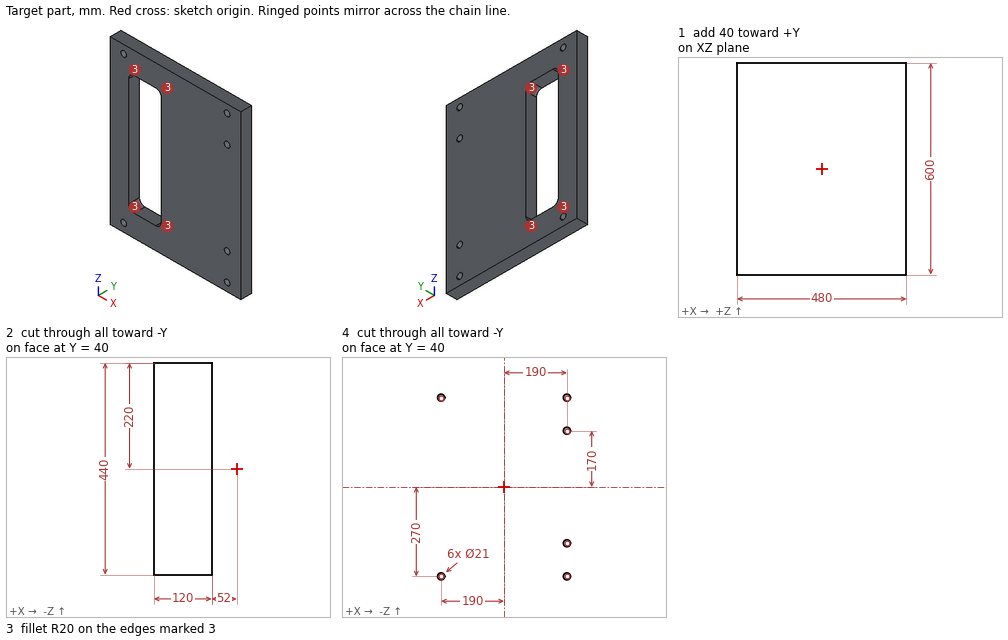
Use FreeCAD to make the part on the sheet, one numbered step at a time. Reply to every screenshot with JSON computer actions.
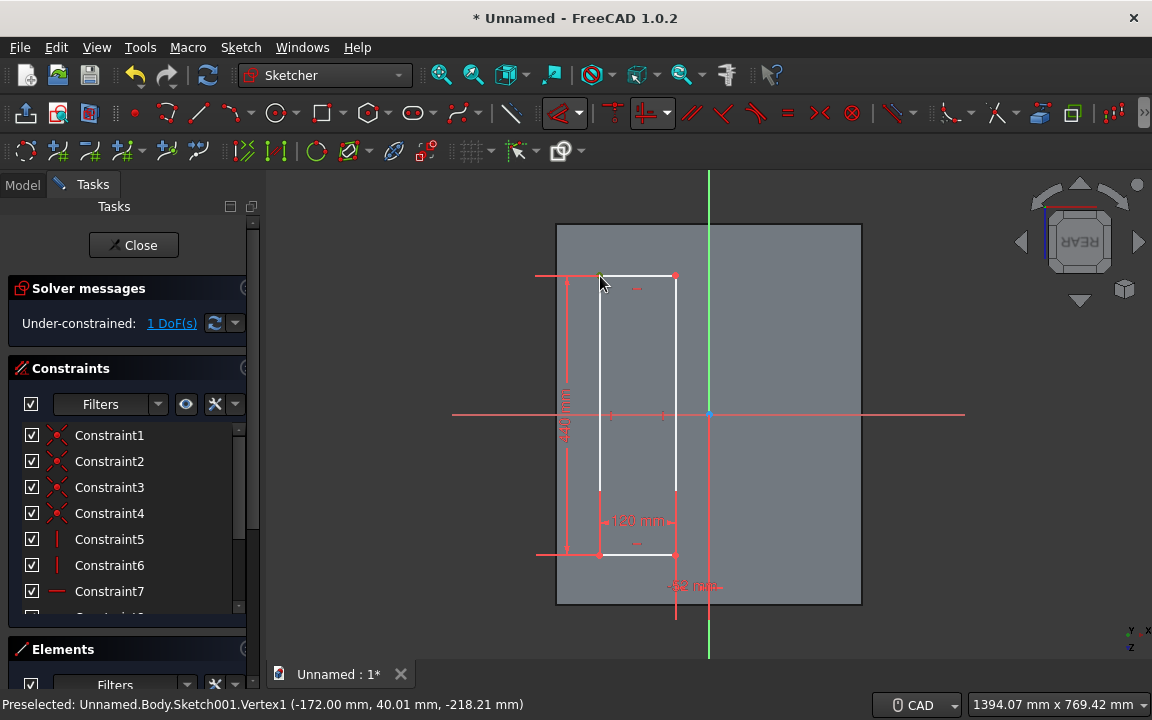
{"action": "left_click", "coordinate": [582, 114]}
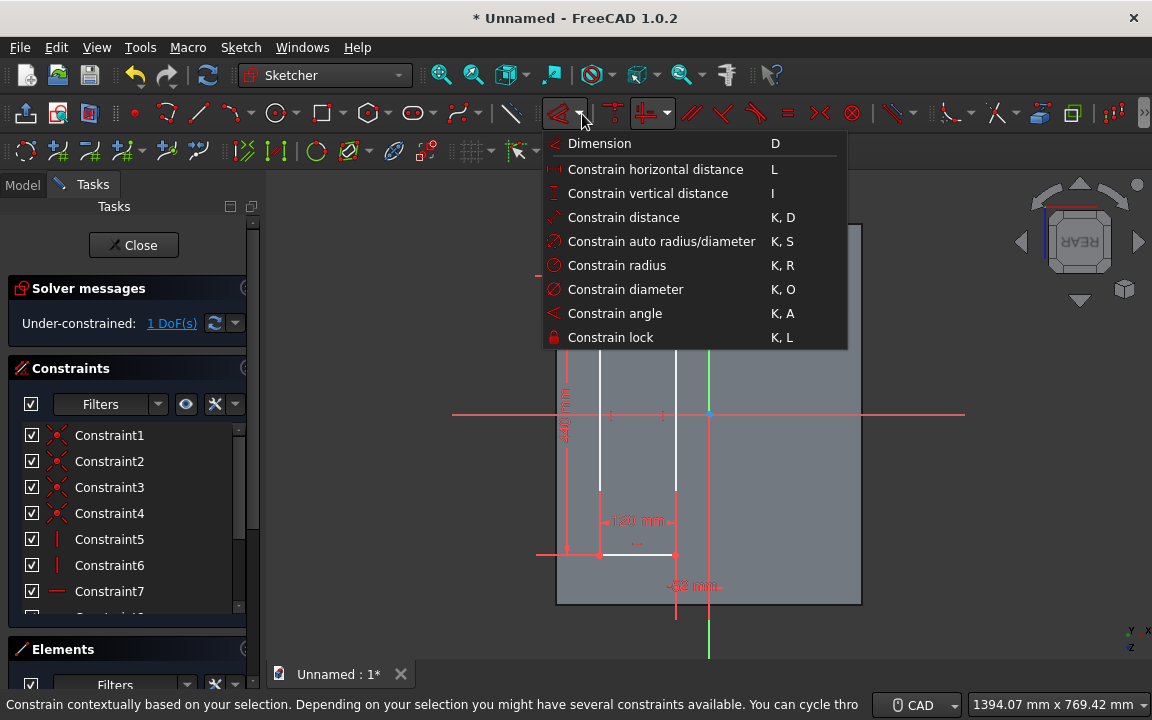
{"action": "left_click", "coordinate": [695, 193]}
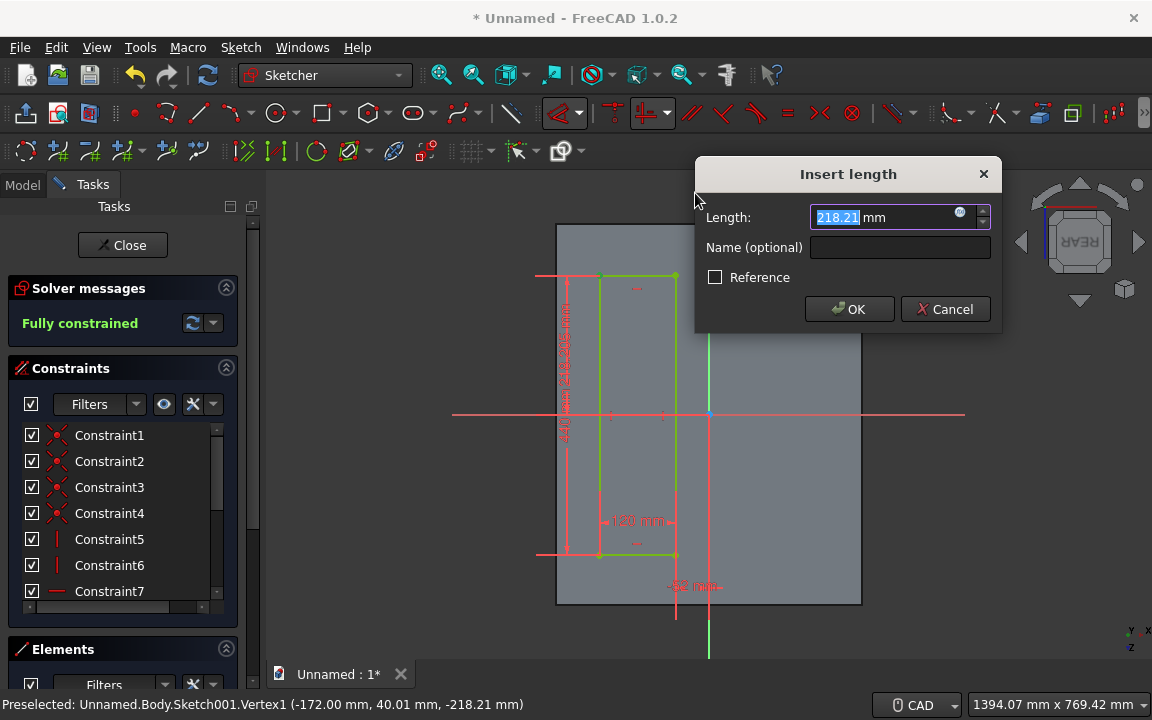
{"action": "type", "text": "220"}
{"action": "key", "text": "Return"}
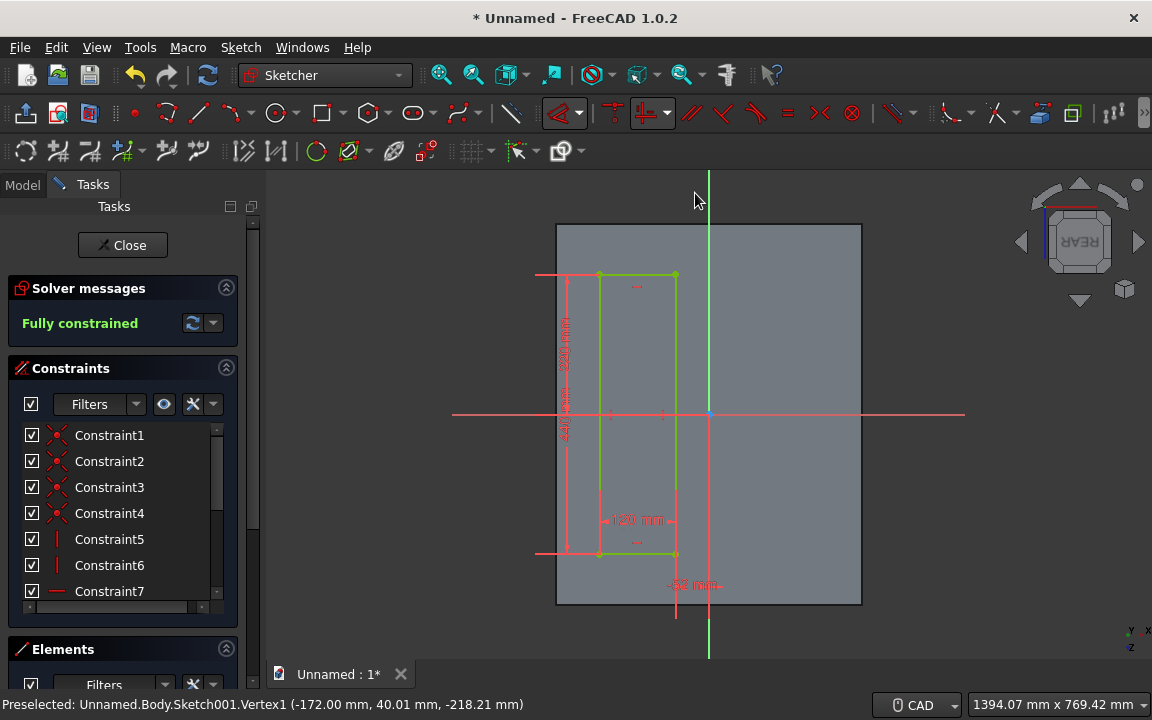
{"action": "left_click", "coordinate": [123, 245]}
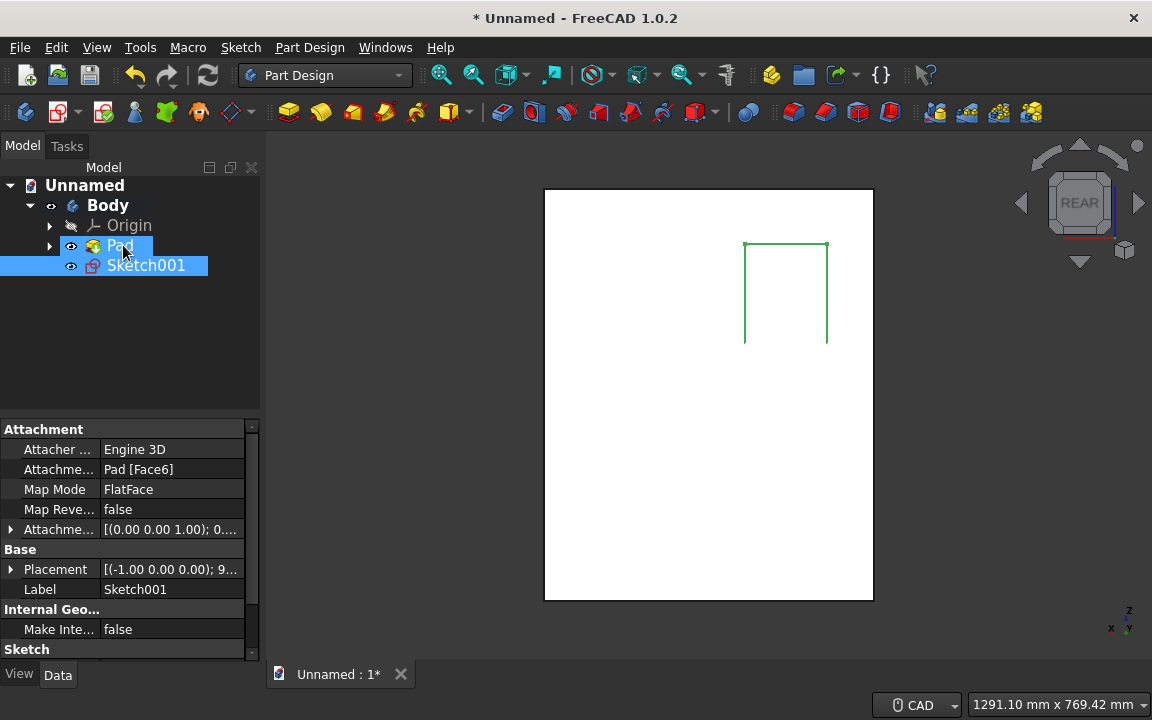
{"action": "left_click", "coordinate": [504, 112]}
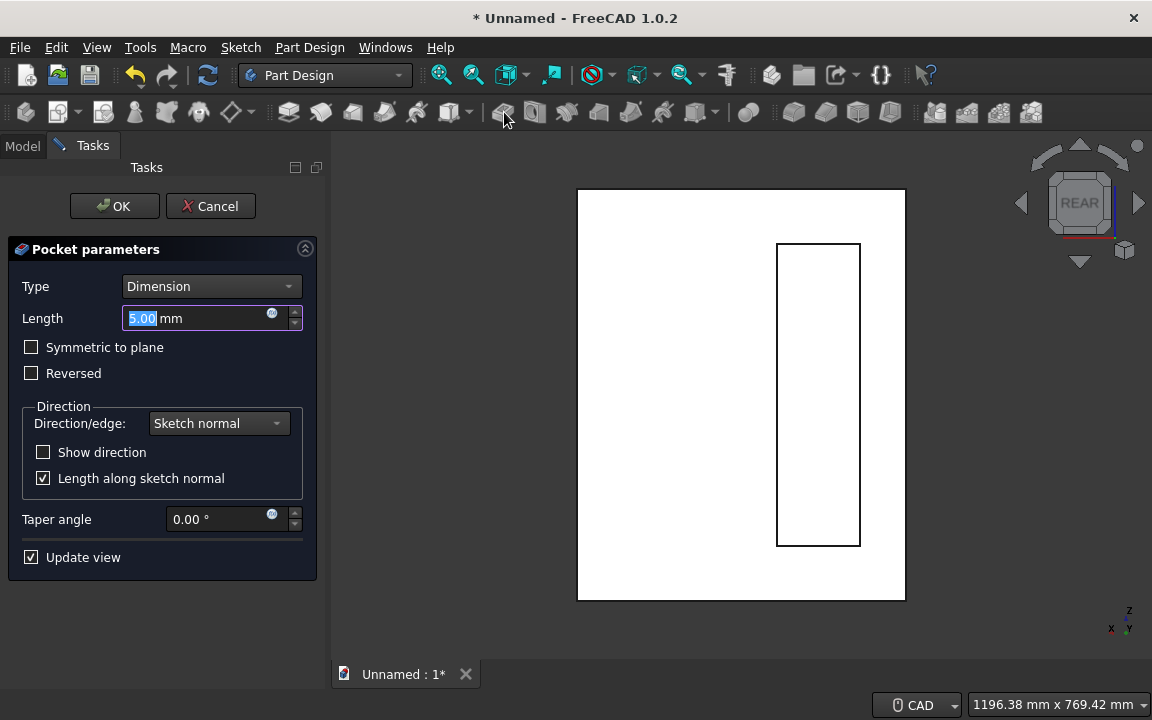
{"action": "left_click", "coordinate": [212, 286]}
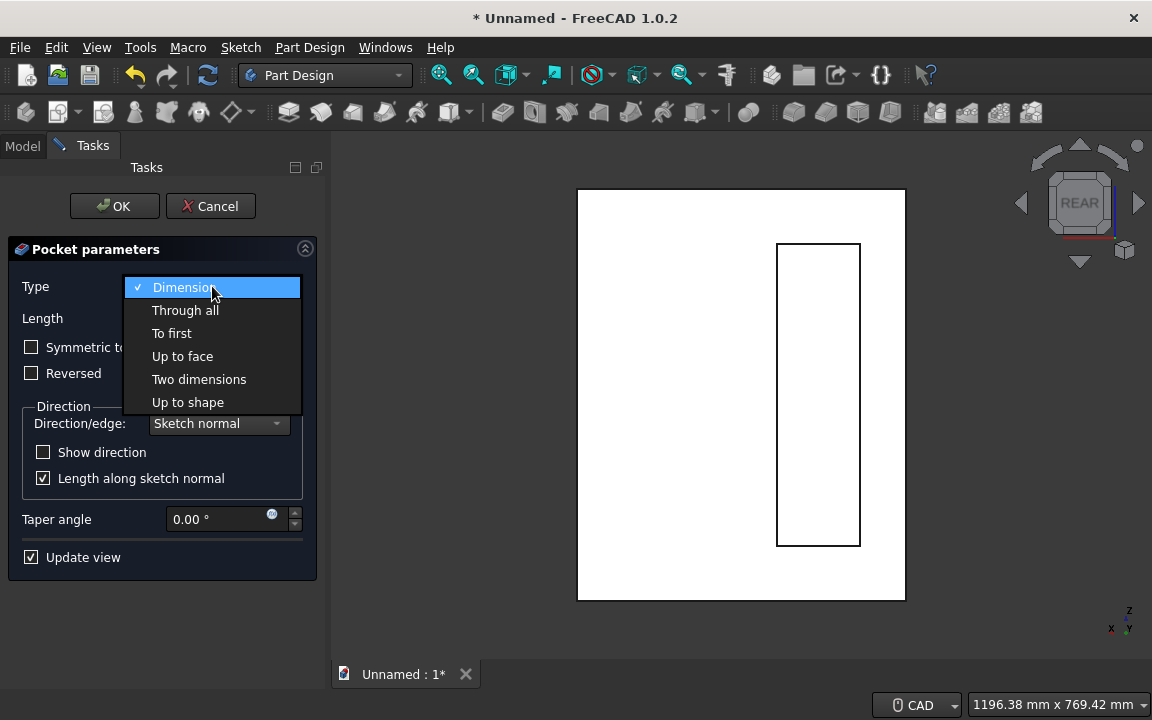
{"action": "left_click", "coordinate": [212, 310]}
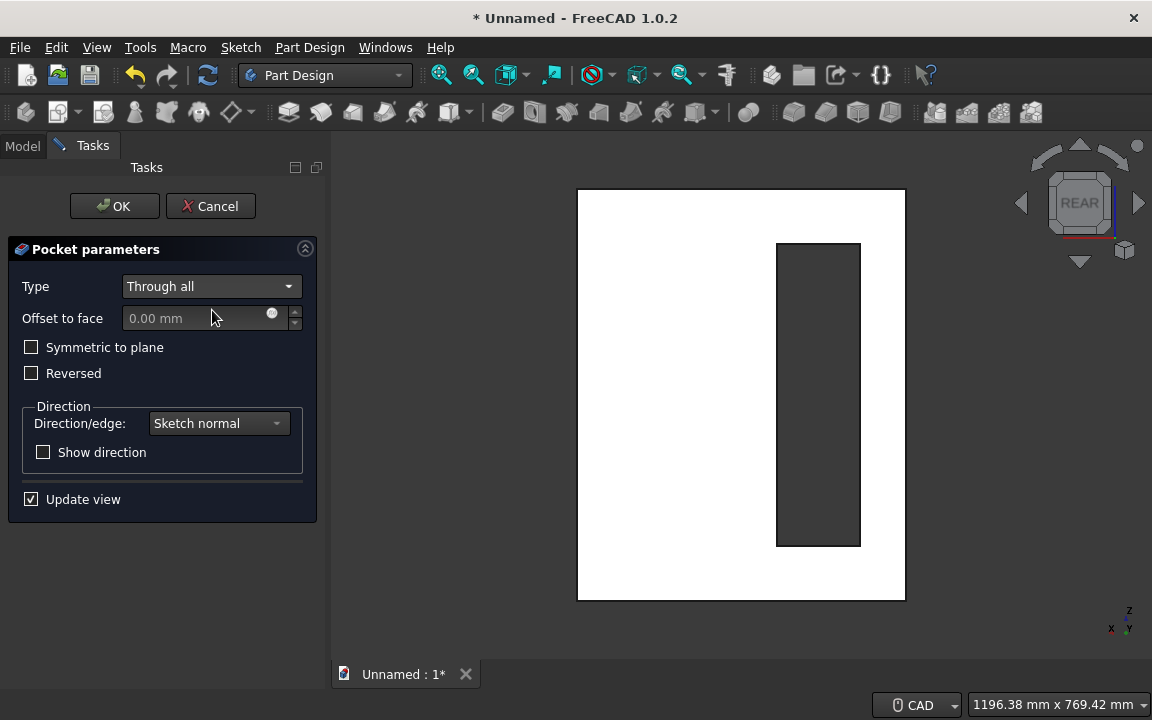
{"action": "left_click", "coordinate": [115, 206]}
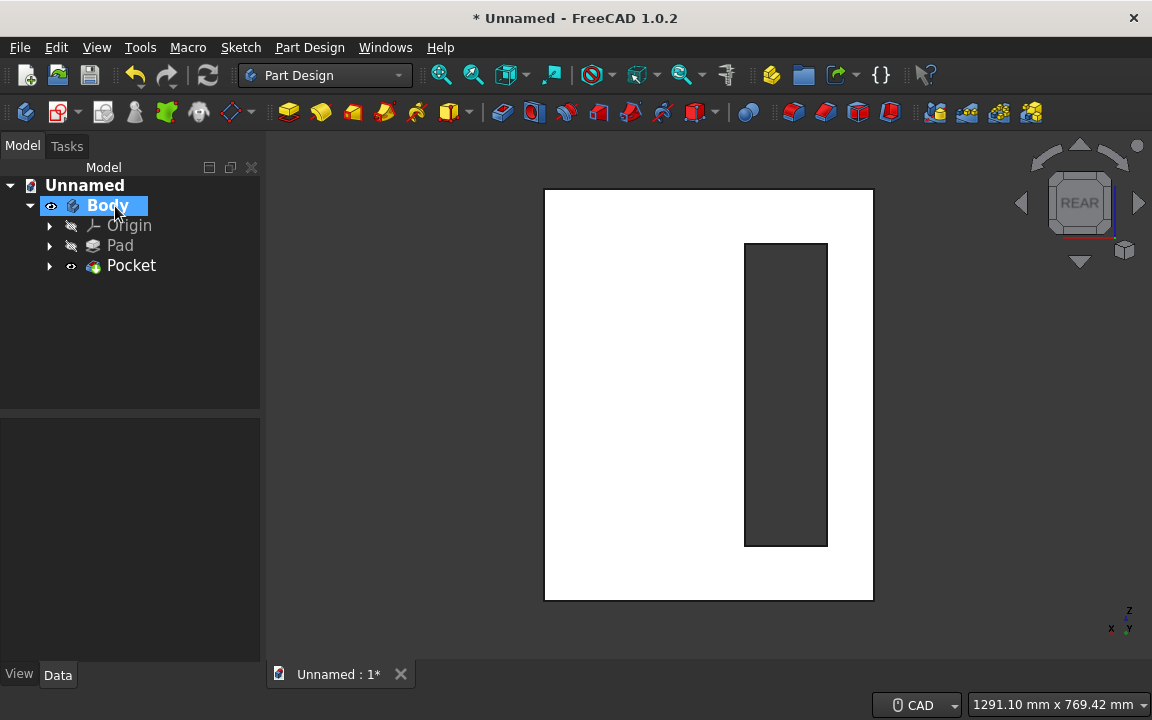
{"action": "key", "text": "0"}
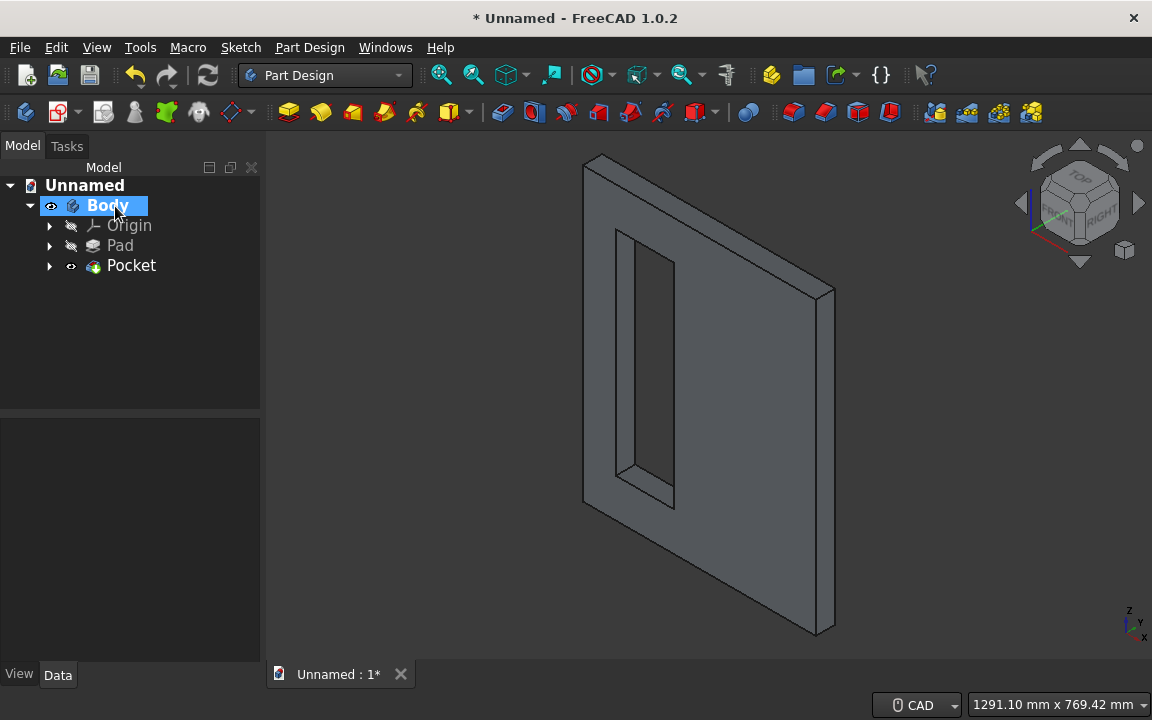
{"action": "key", "text": "2"}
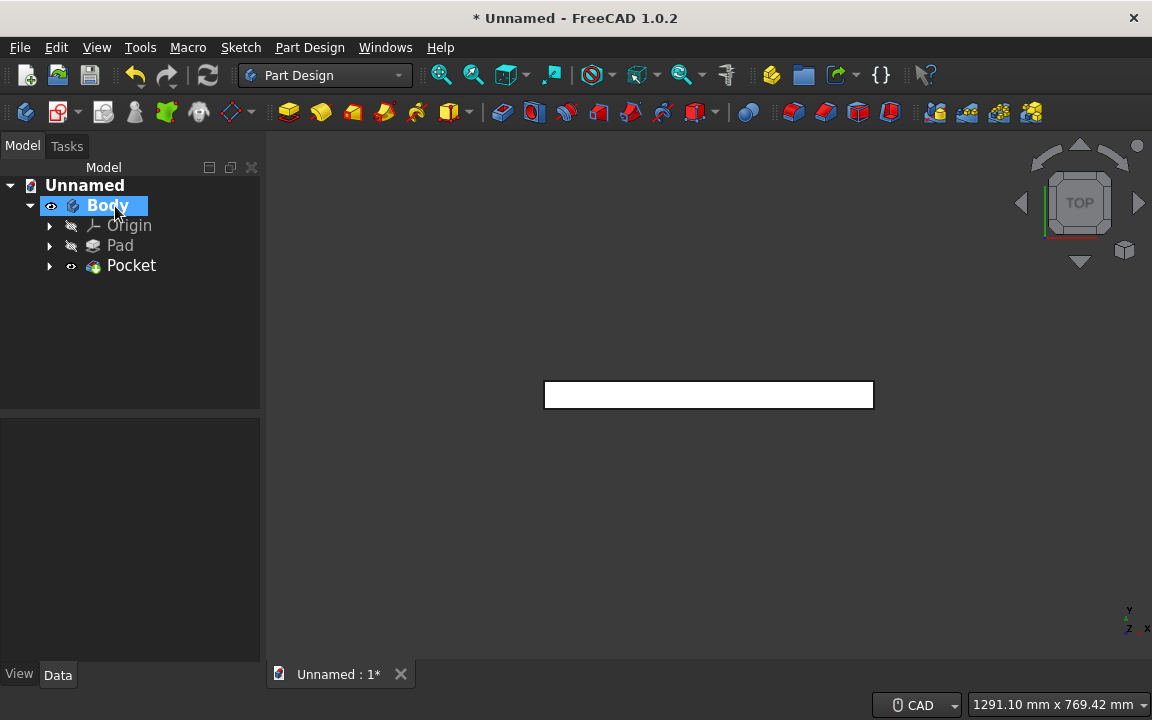
{"action": "left_click", "coordinate": [442, 76]}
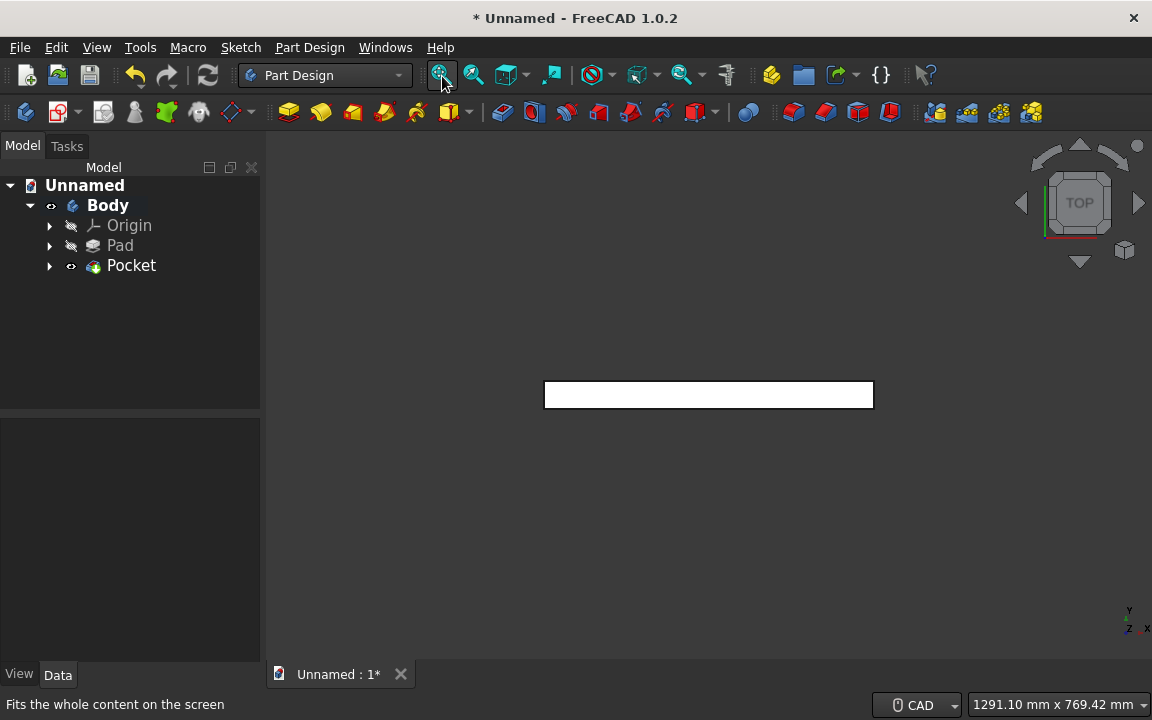
{"action": "key", "text": "1"}